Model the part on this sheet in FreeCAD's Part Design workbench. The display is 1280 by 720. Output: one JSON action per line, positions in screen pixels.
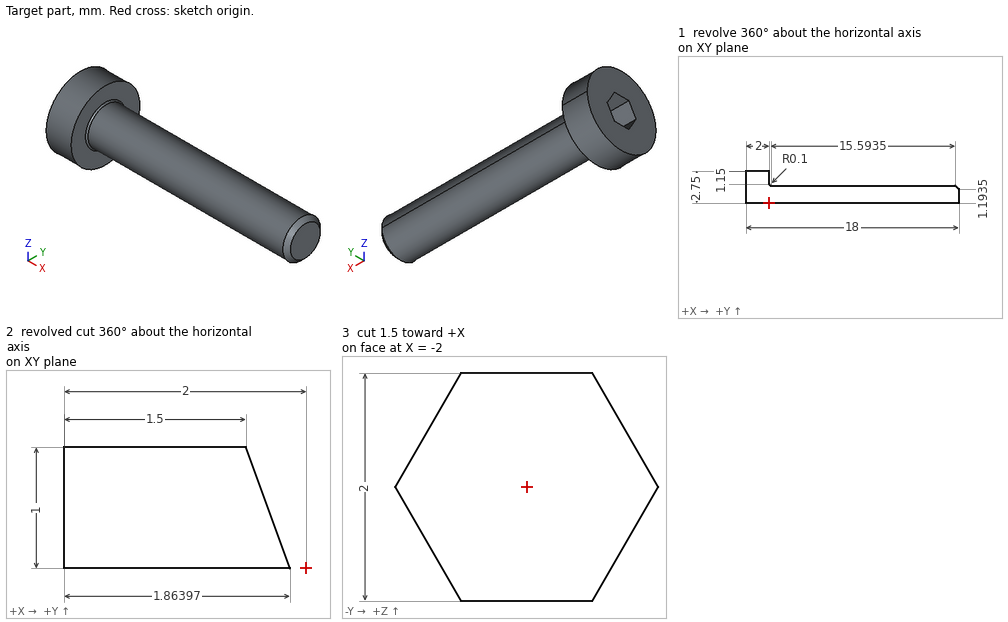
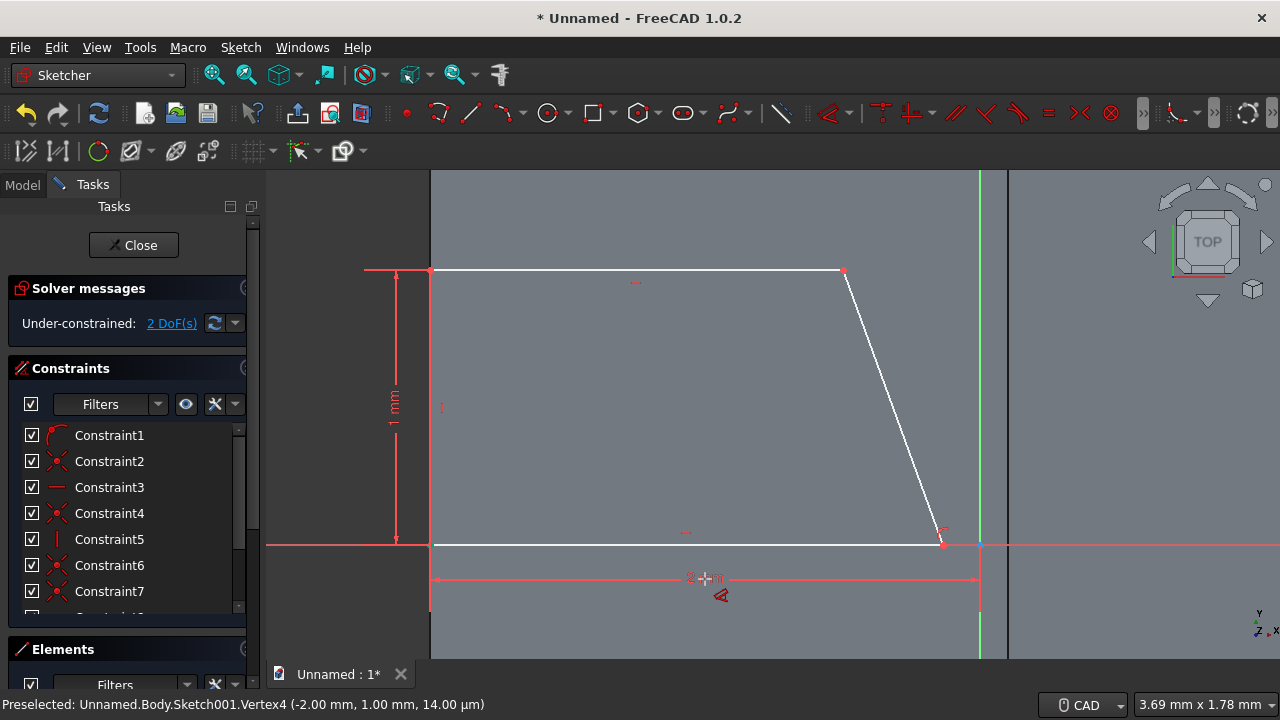
{"action": "left_click", "coordinate": [719, 270]}
{"action": "left_click", "coordinate": [637, 236]}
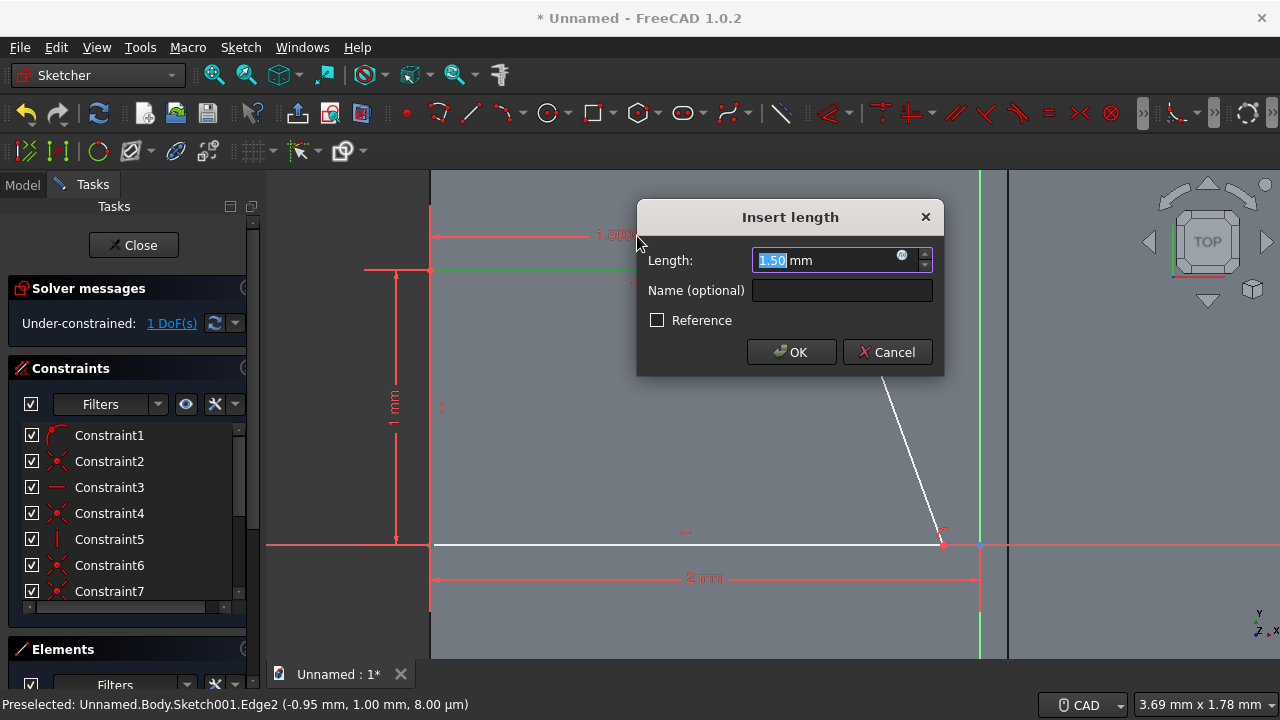
{"action": "type", "text": "1.5"}
{"action": "key", "text": "Return"}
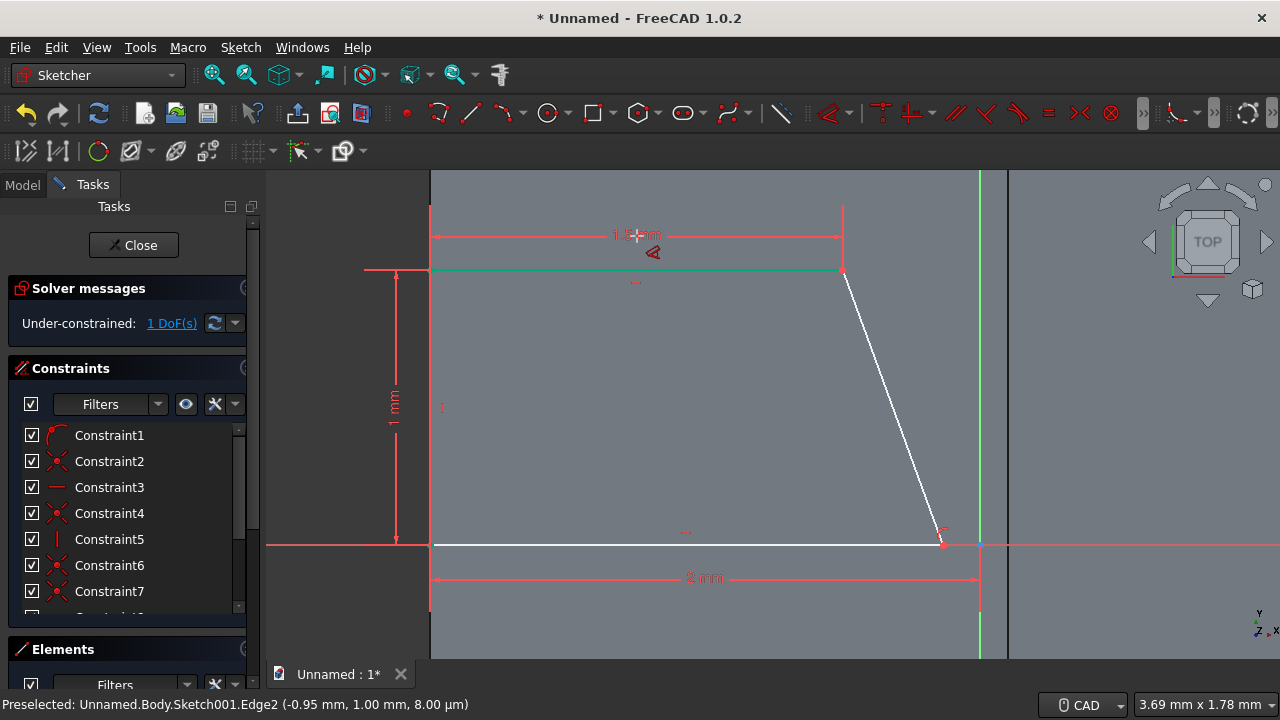
{"action": "left_click", "coordinate": [584, 545]}
{"action": "left_click", "coordinate": [569, 579]}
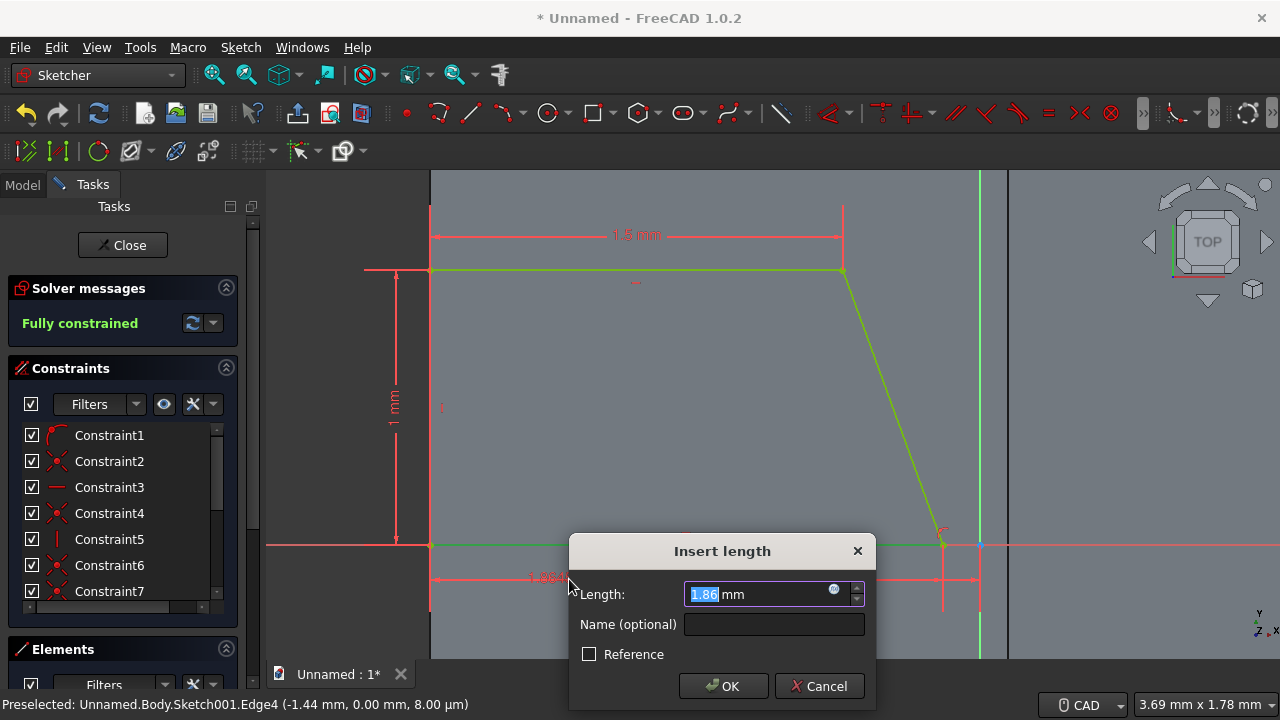
{"action": "type", "text": "1.86397"}
{"action": "key", "text": "Return"}
{"action": "key", "text": "Escape"}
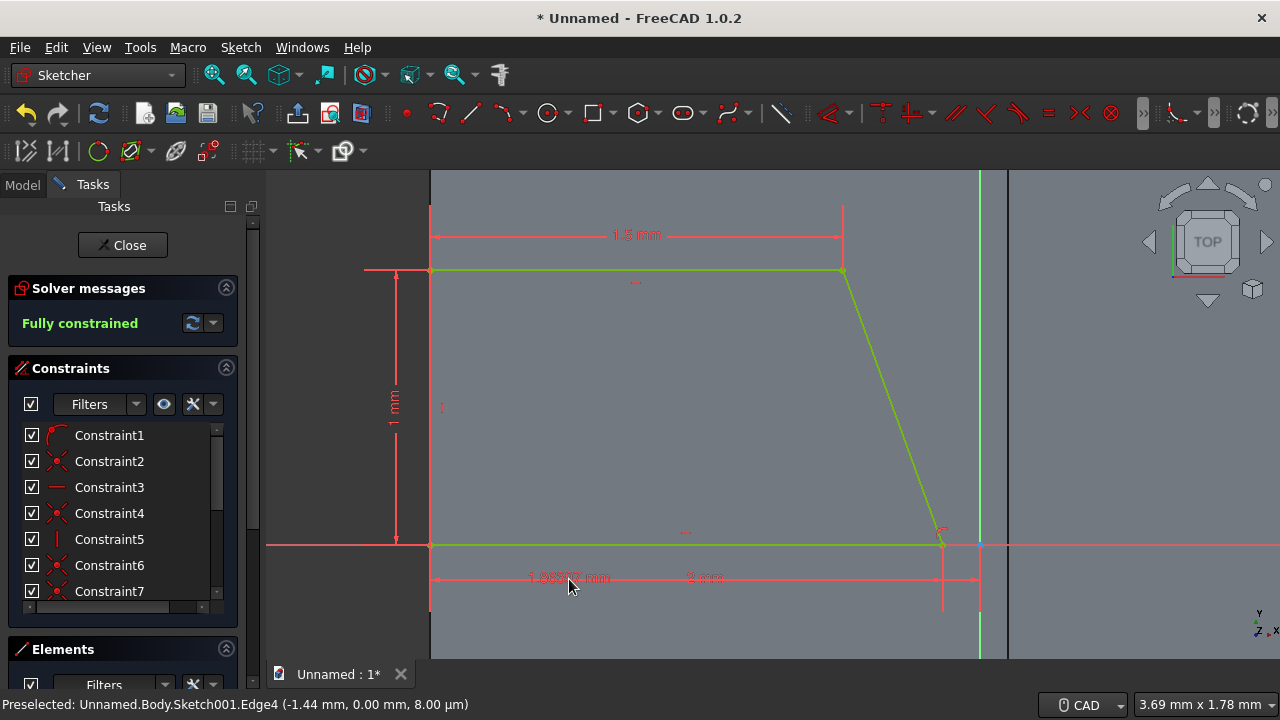
{"action": "left_click", "coordinate": [123, 245]}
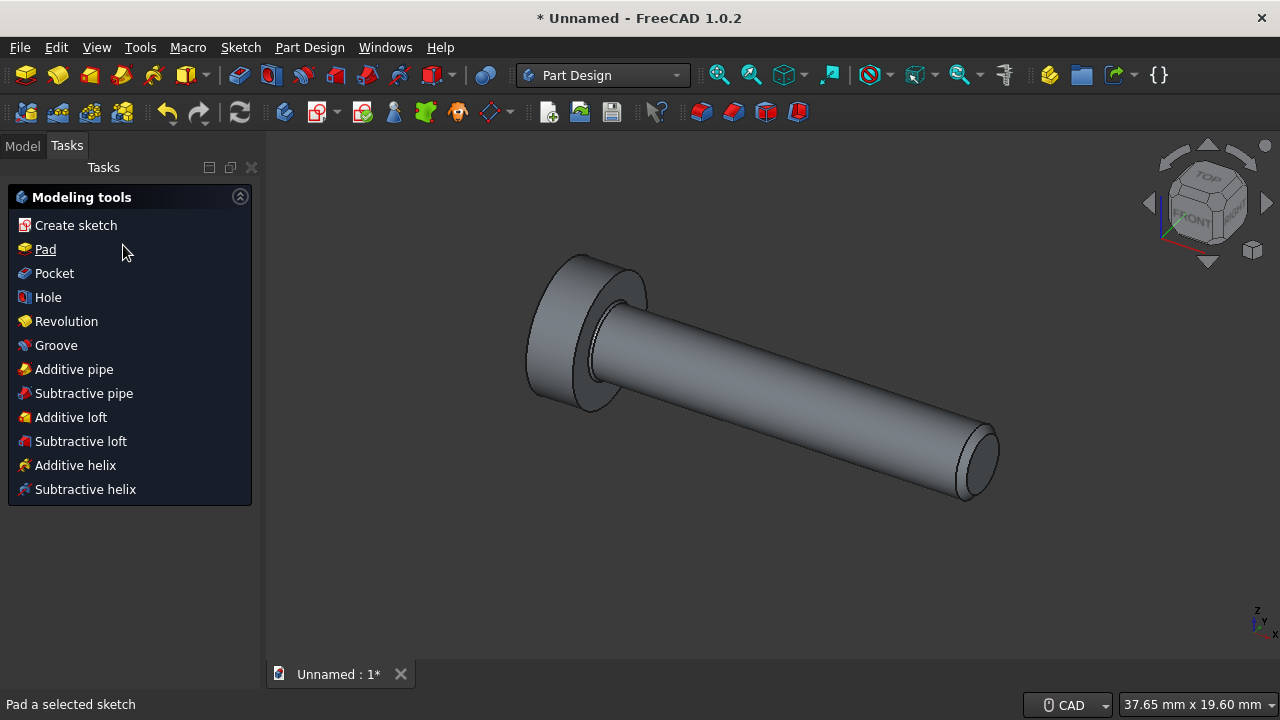
{"action": "left_click", "coordinate": [304, 76]}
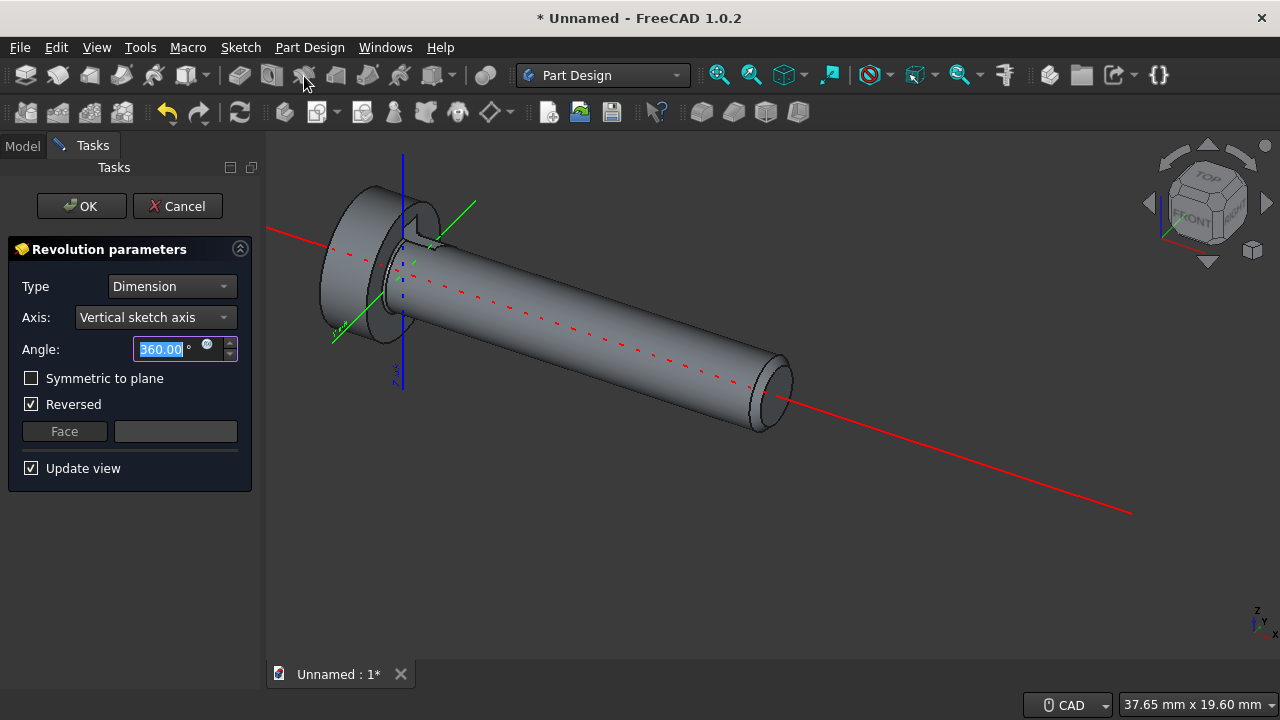
{"action": "left_click", "coordinate": [156, 318]}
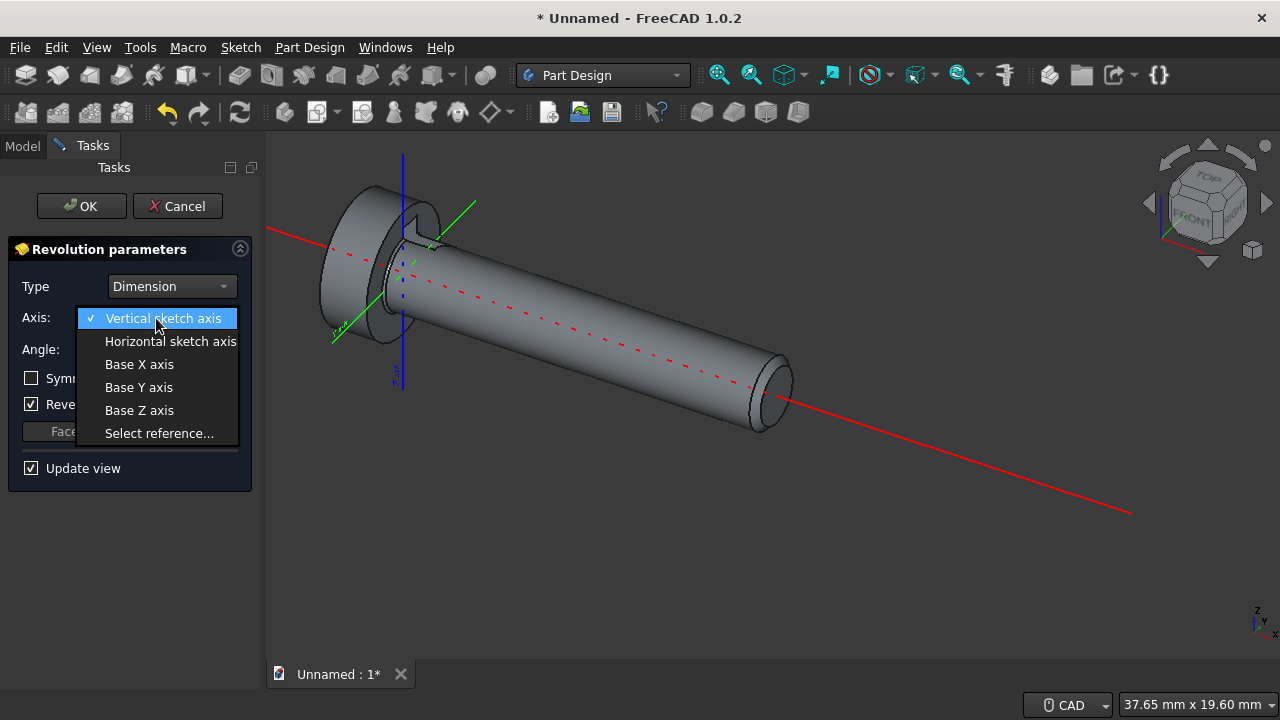
{"action": "left_click", "coordinate": [156, 342]}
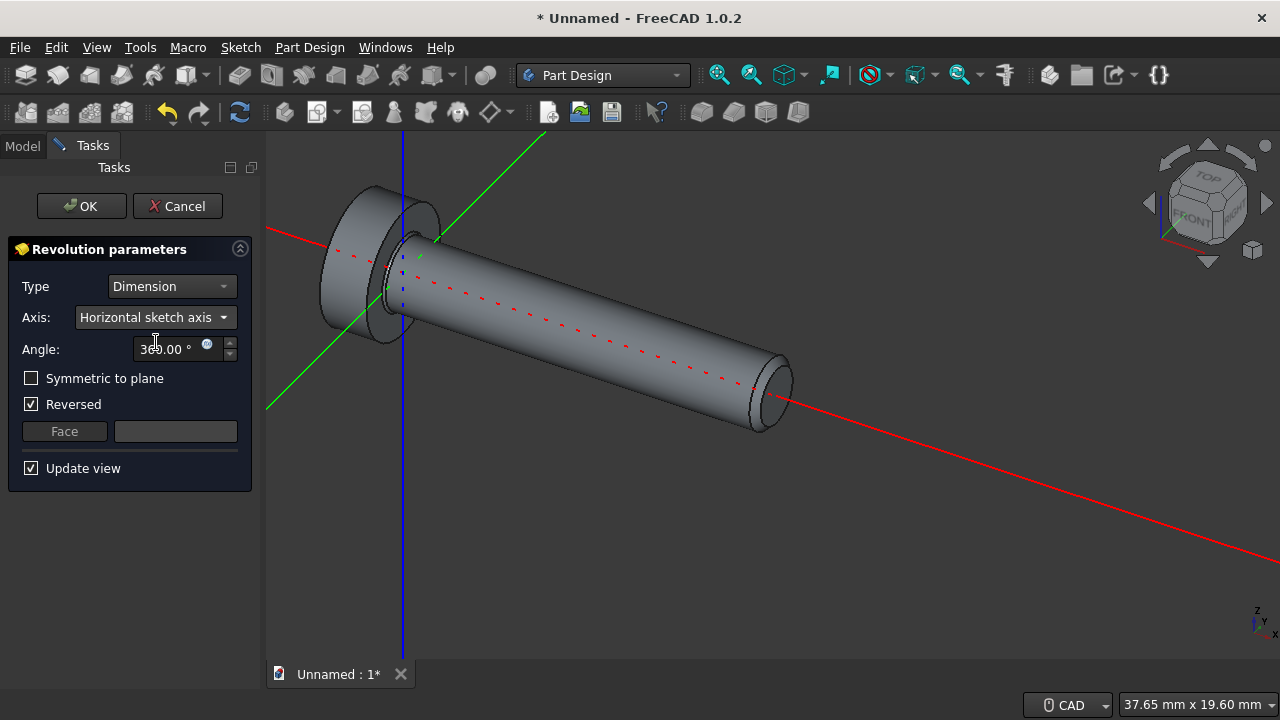
{"action": "left_click", "coordinate": [82, 206]}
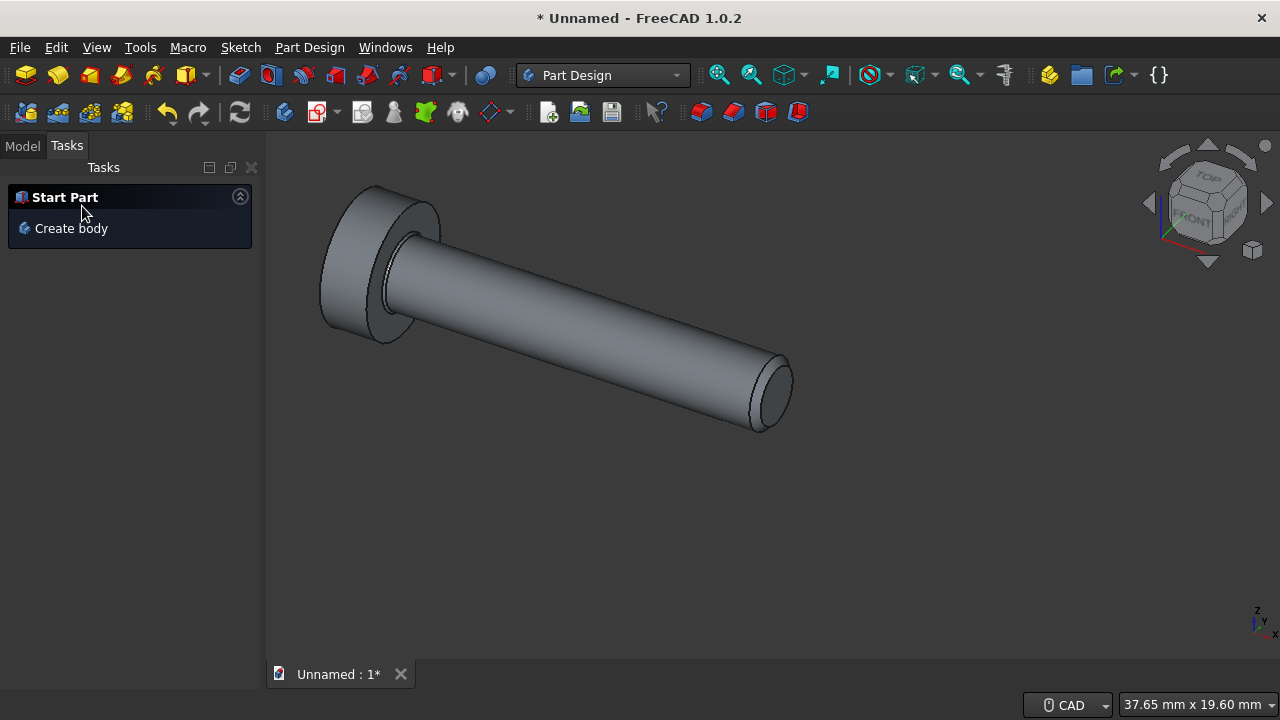
{"action": "key", "text": "6"}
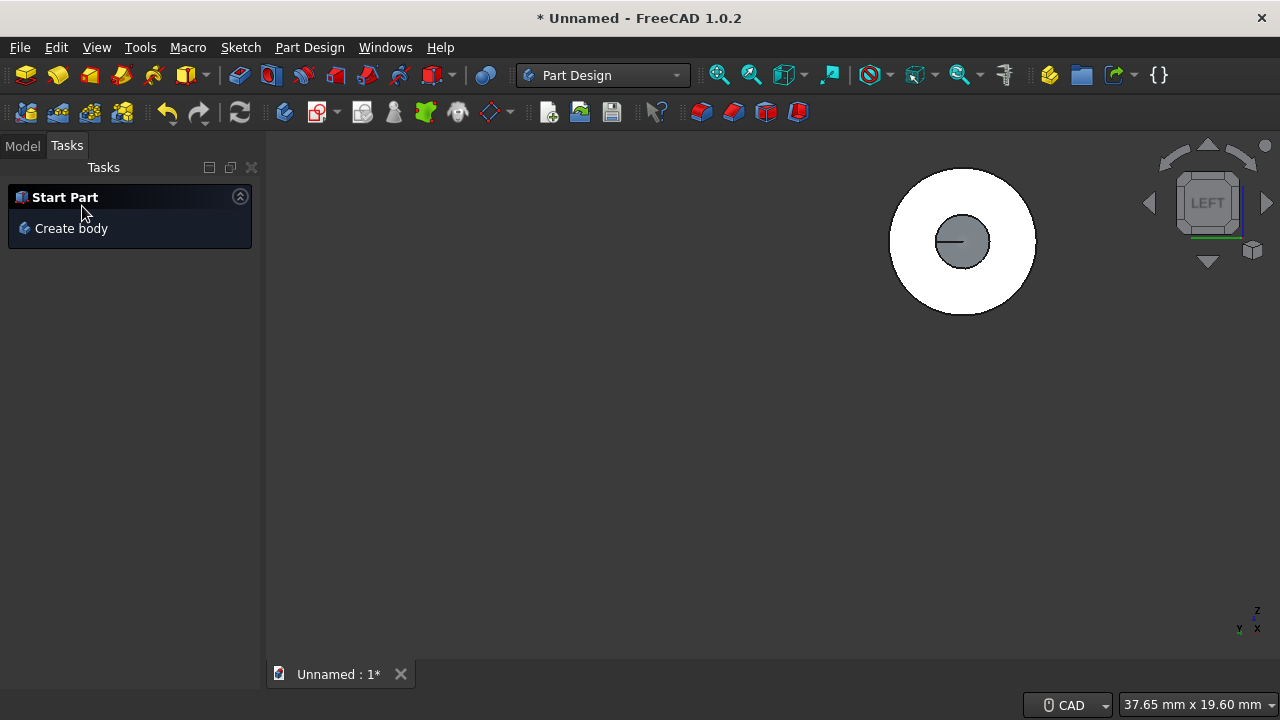
{"action": "left_click", "coordinate": [720, 76]}